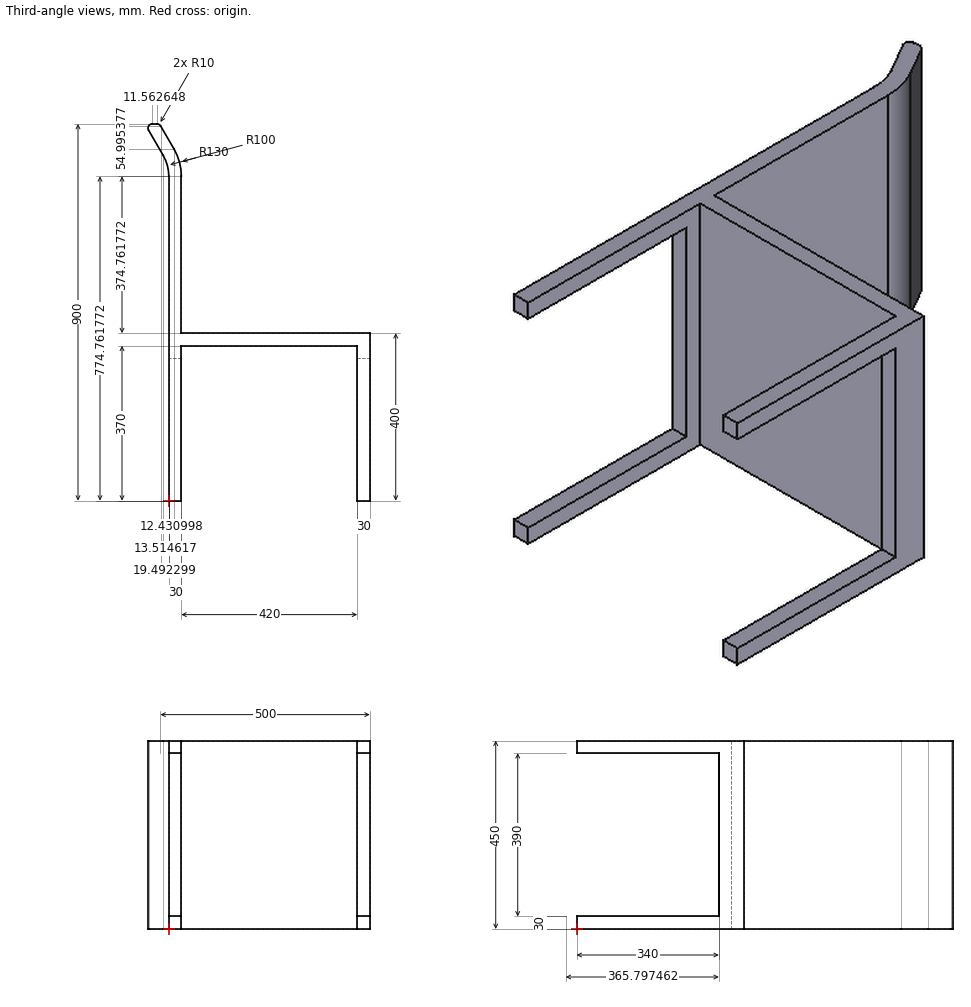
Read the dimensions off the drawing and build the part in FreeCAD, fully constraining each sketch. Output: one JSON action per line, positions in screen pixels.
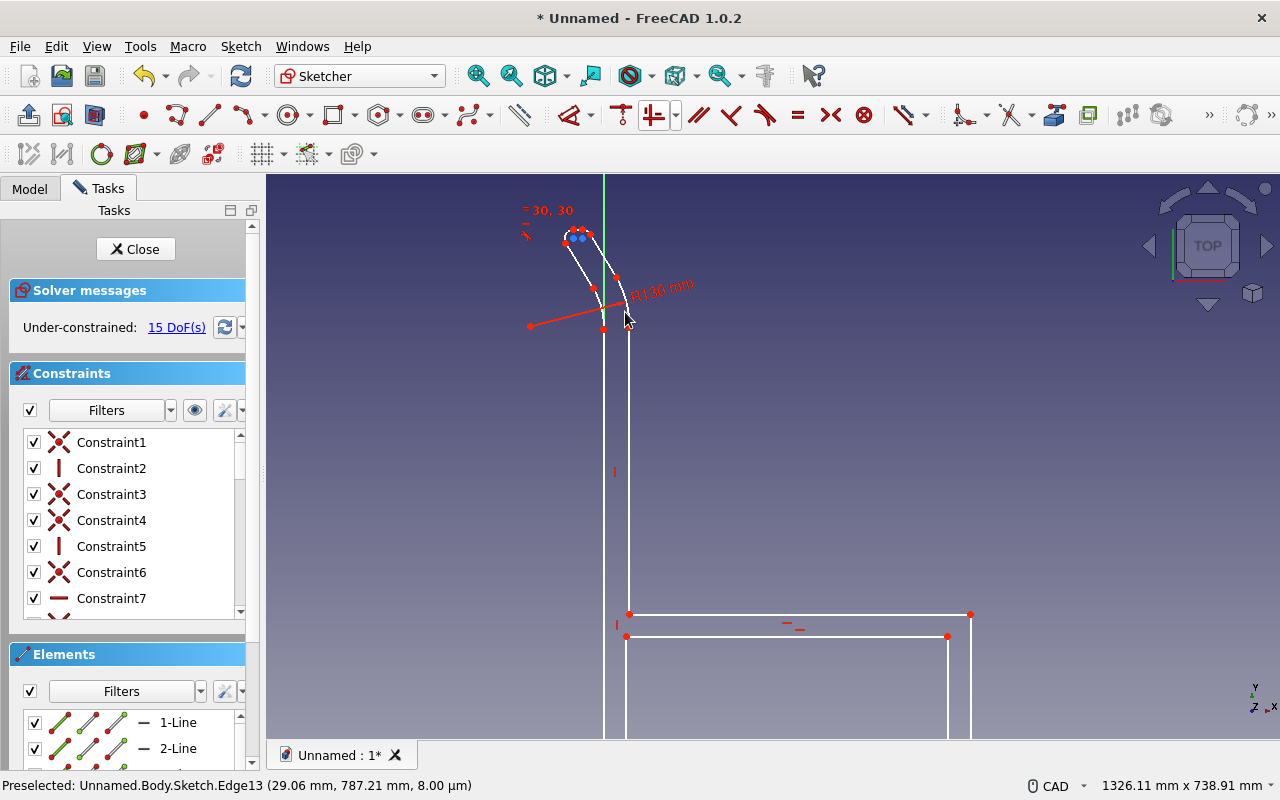
{"action": "scroll", "coordinate": [587, 231], "scroll_direction": "up", "scroll_amount": 9}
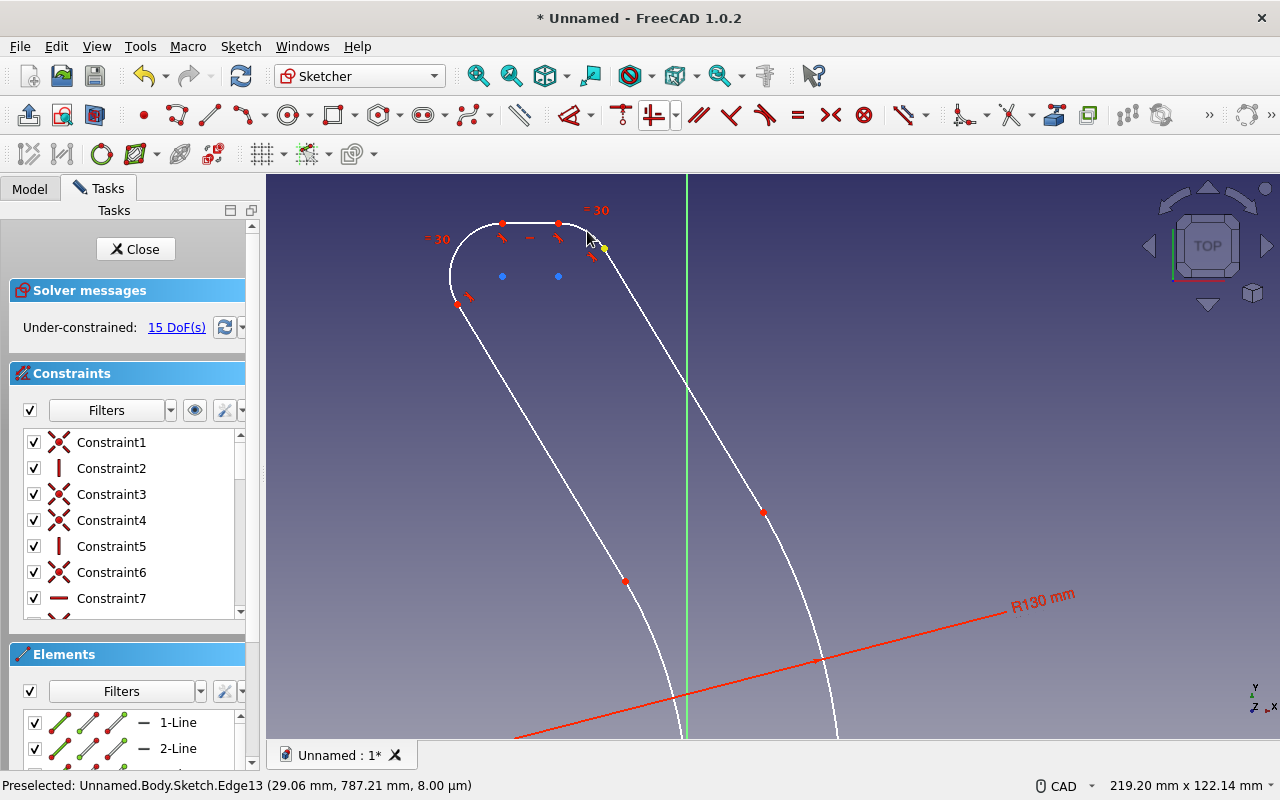
{"action": "left_click", "coordinate": [585, 230]}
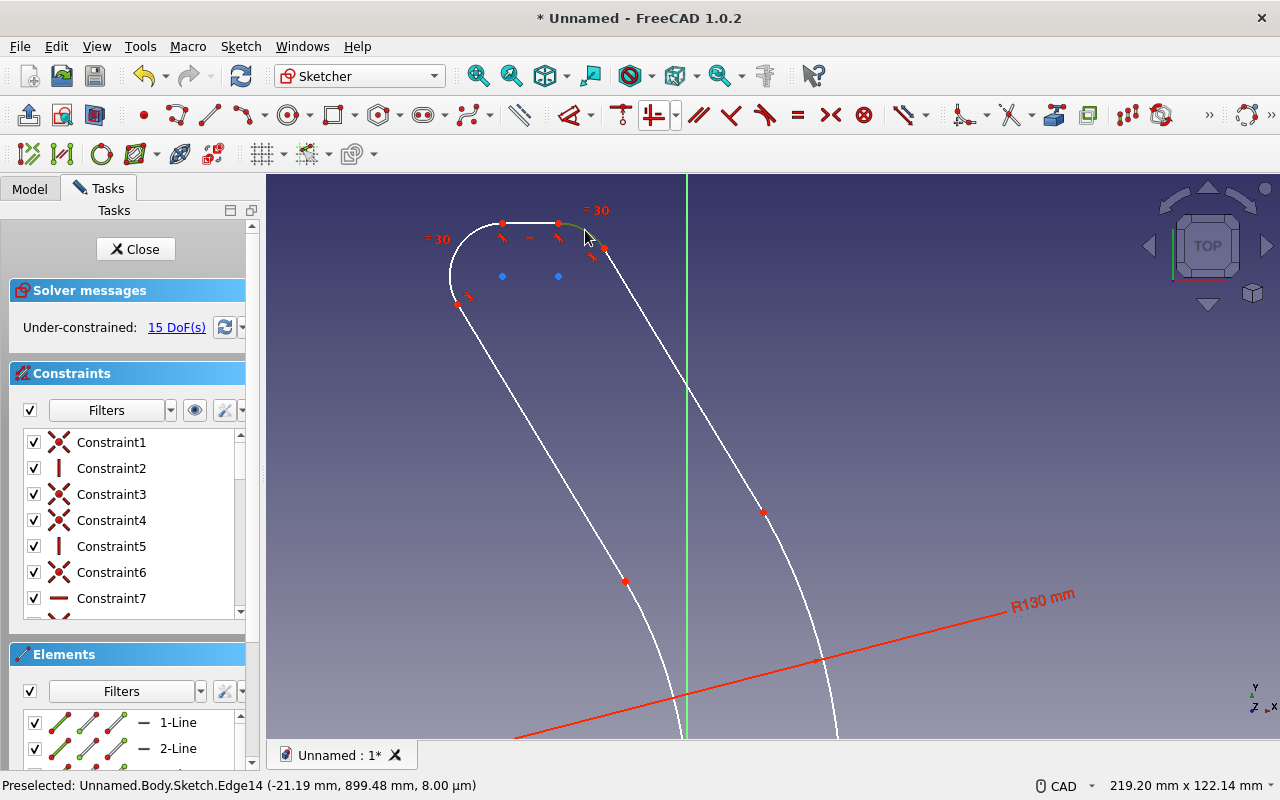
{"action": "left_click", "coordinate": [590, 116]}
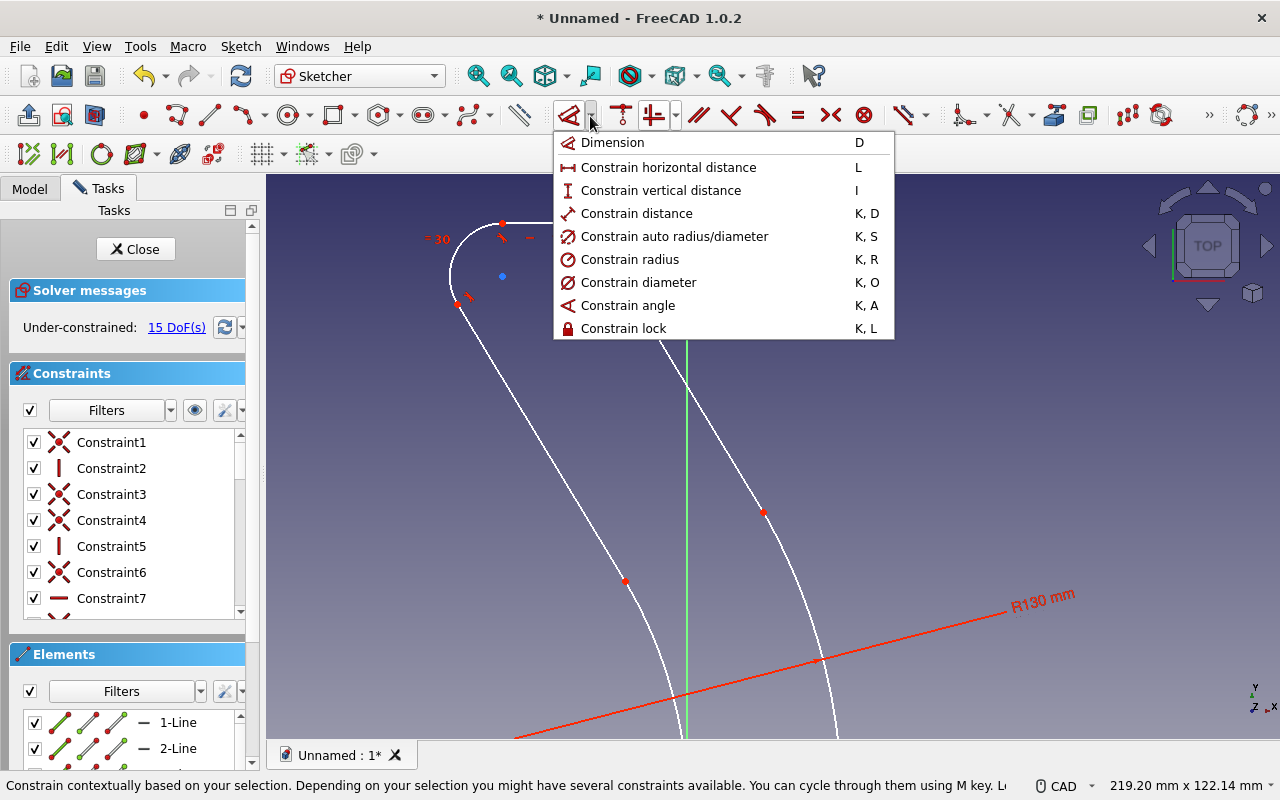
{"action": "left_click", "coordinate": [724, 260]}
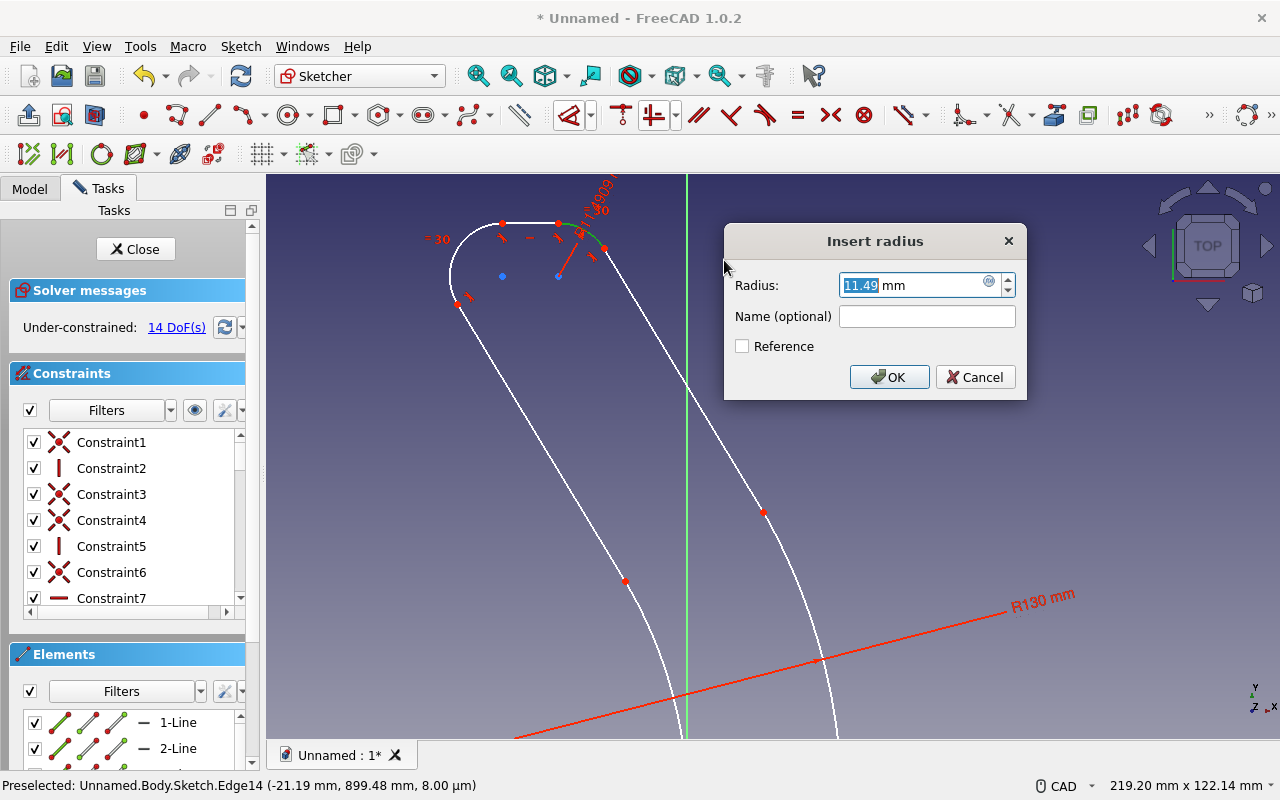
{"action": "type", "text": "10"}
{"action": "key", "text": "Return"}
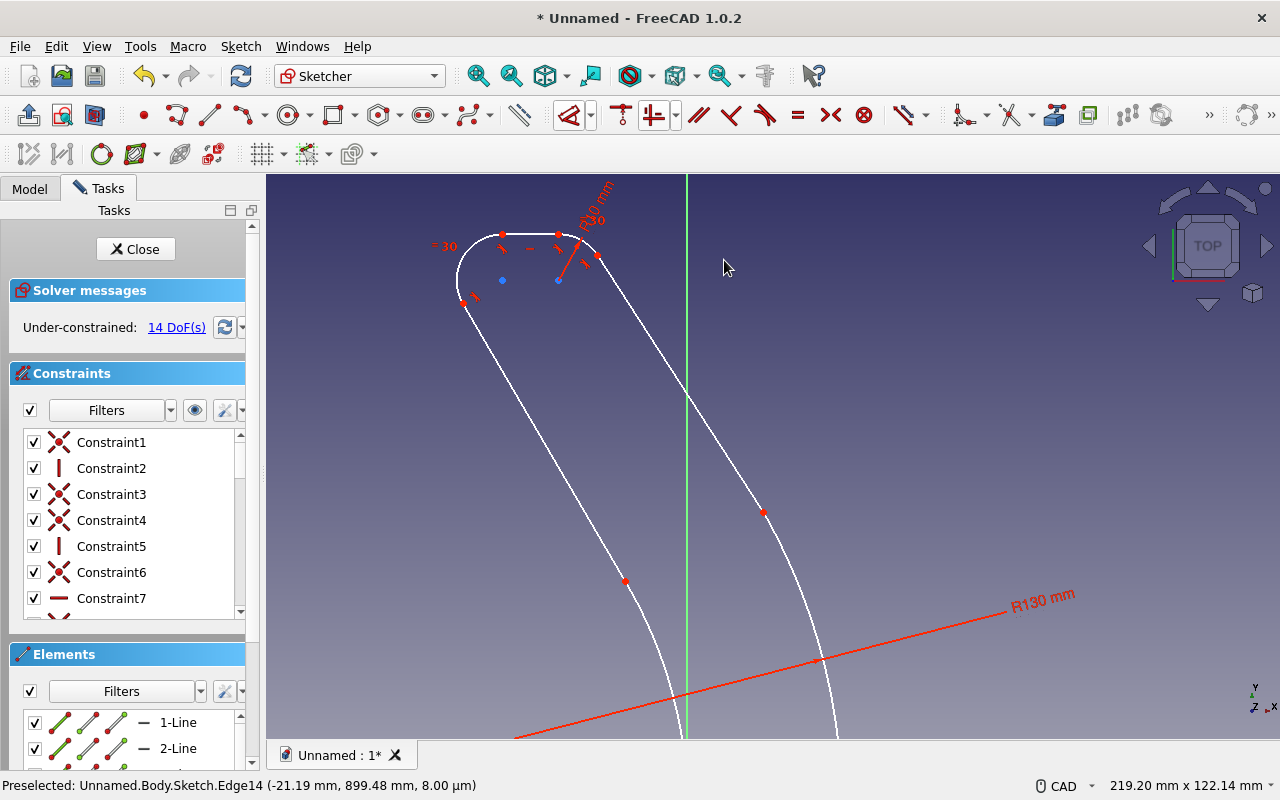
{"action": "left_click", "coordinate": [658, 650]}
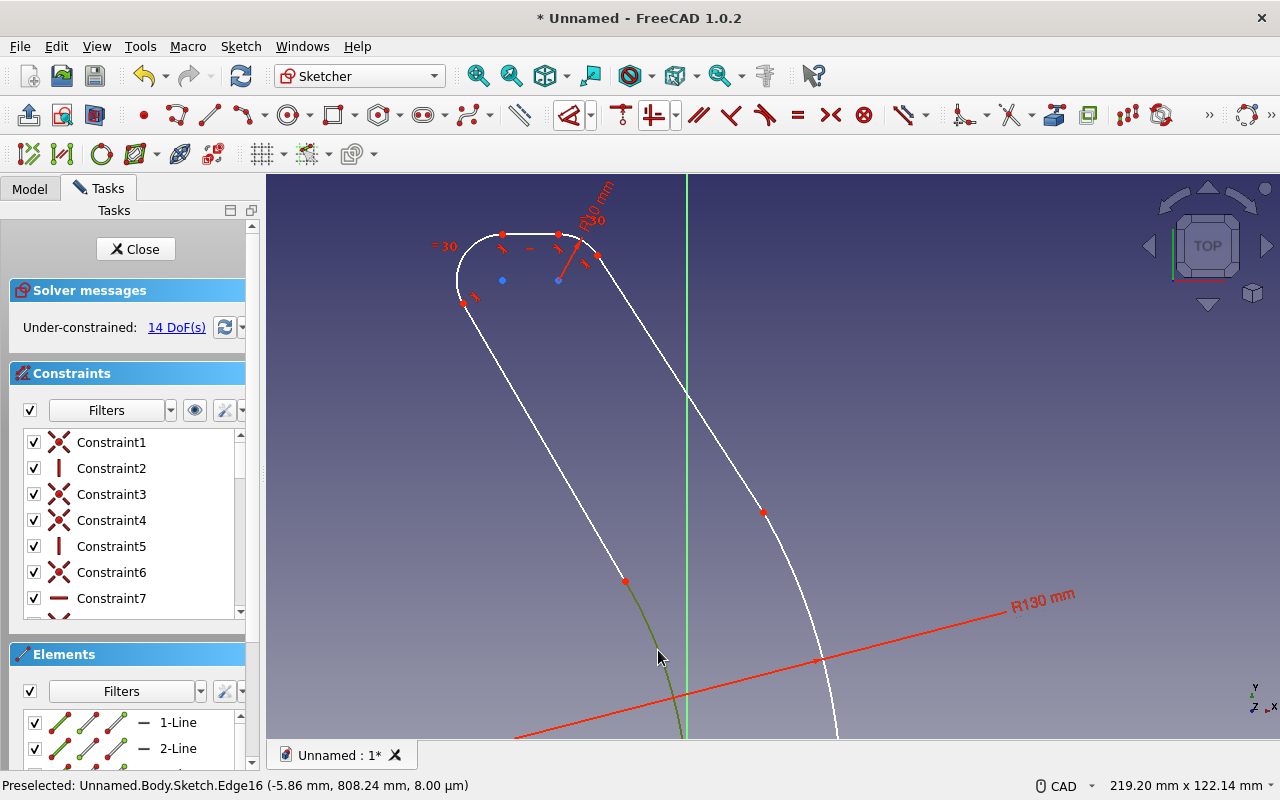
{"action": "left_click", "coordinate": [590, 116]}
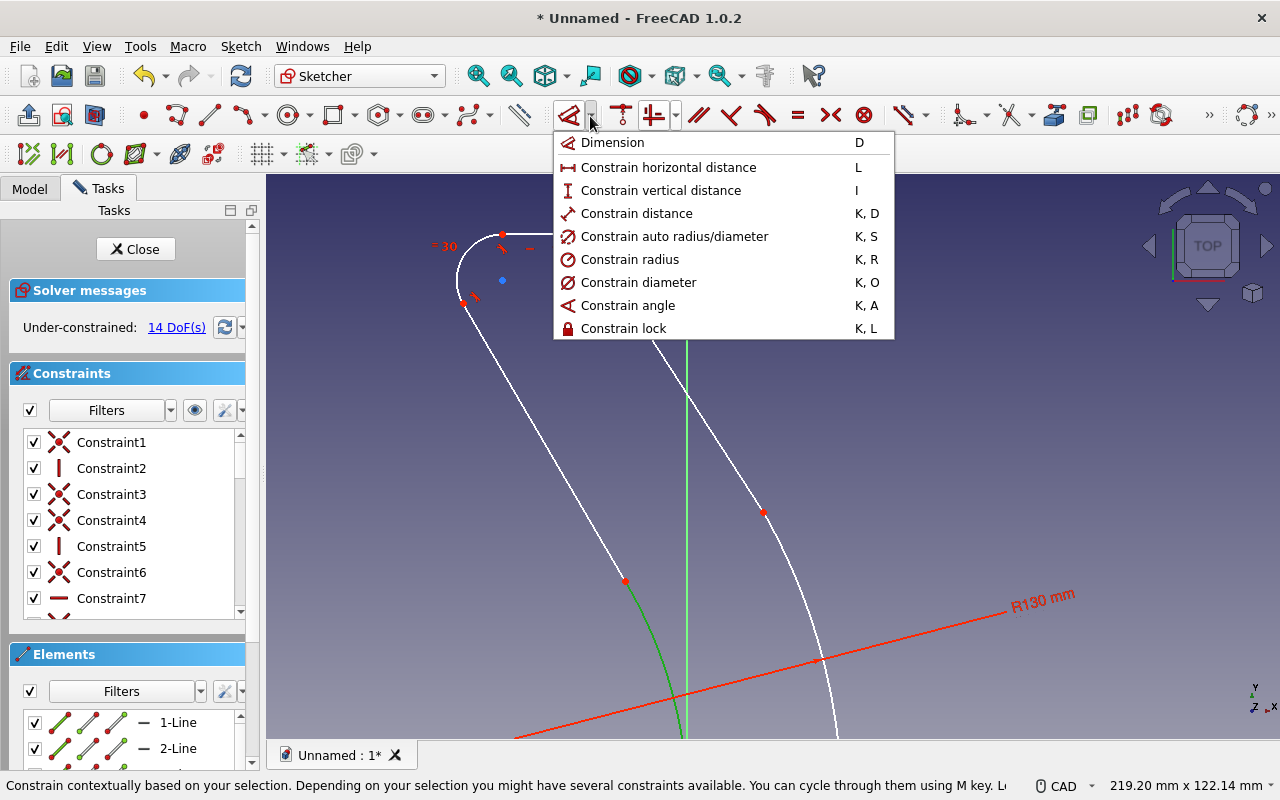
{"action": "left_click", "coordinate": [724, 260]}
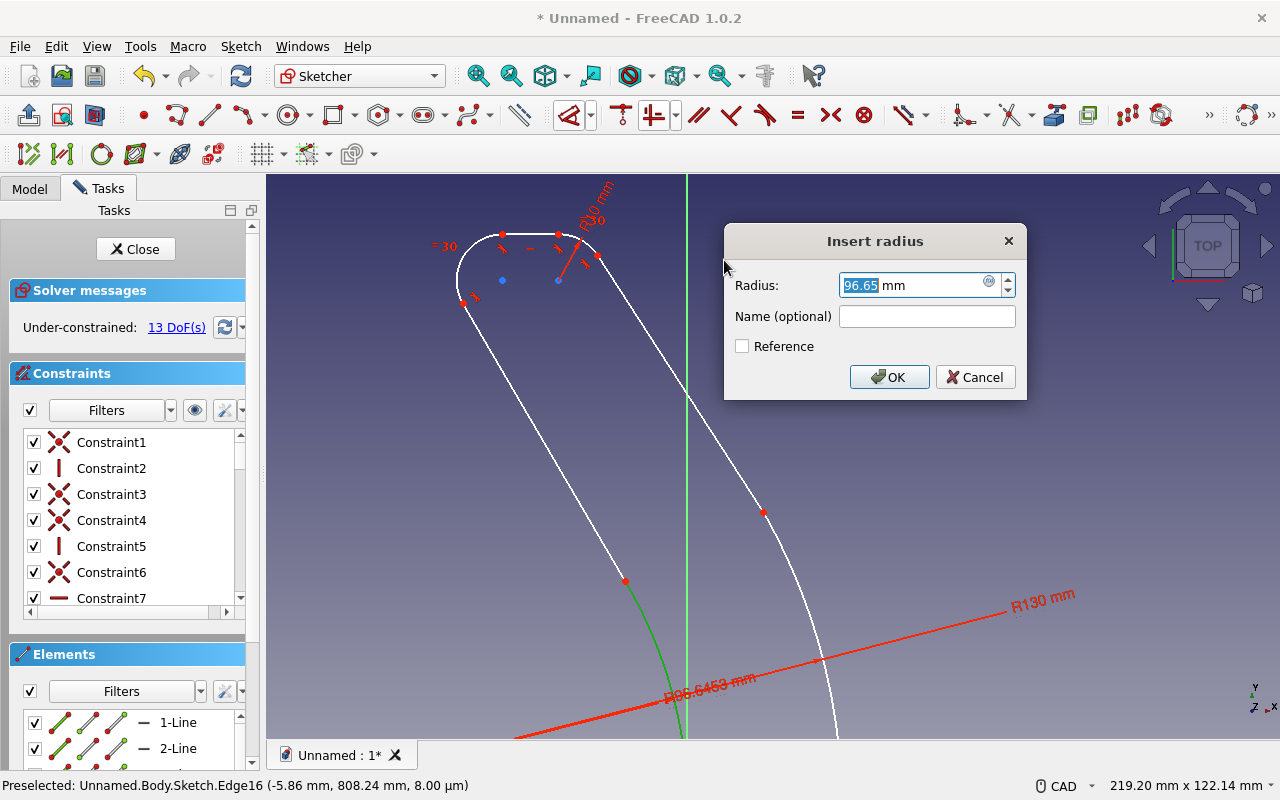
{"action": "type", "text": "100"}
{"action": "key", "text": "Return"}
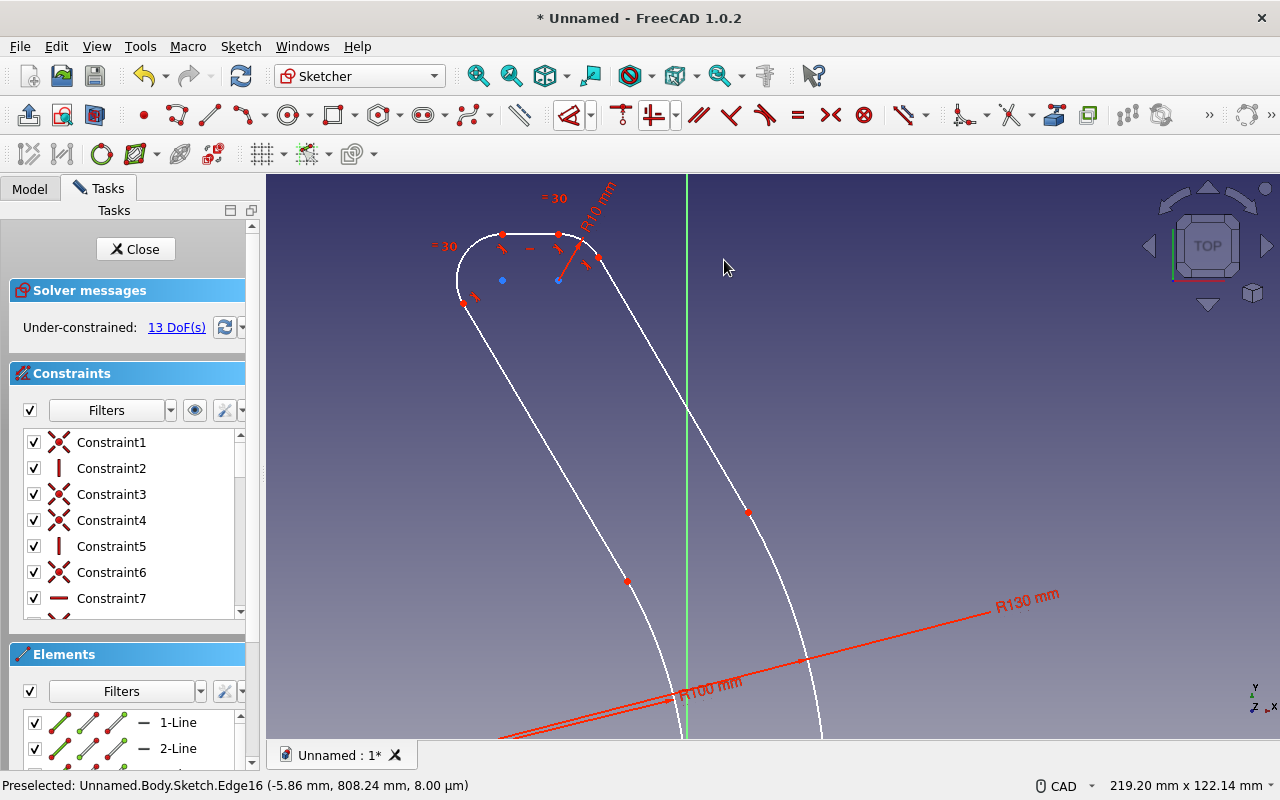
{"action": "scroll", "coordinate": [607, 271], "scroll_direction": "down", "scroll_amount": 12}